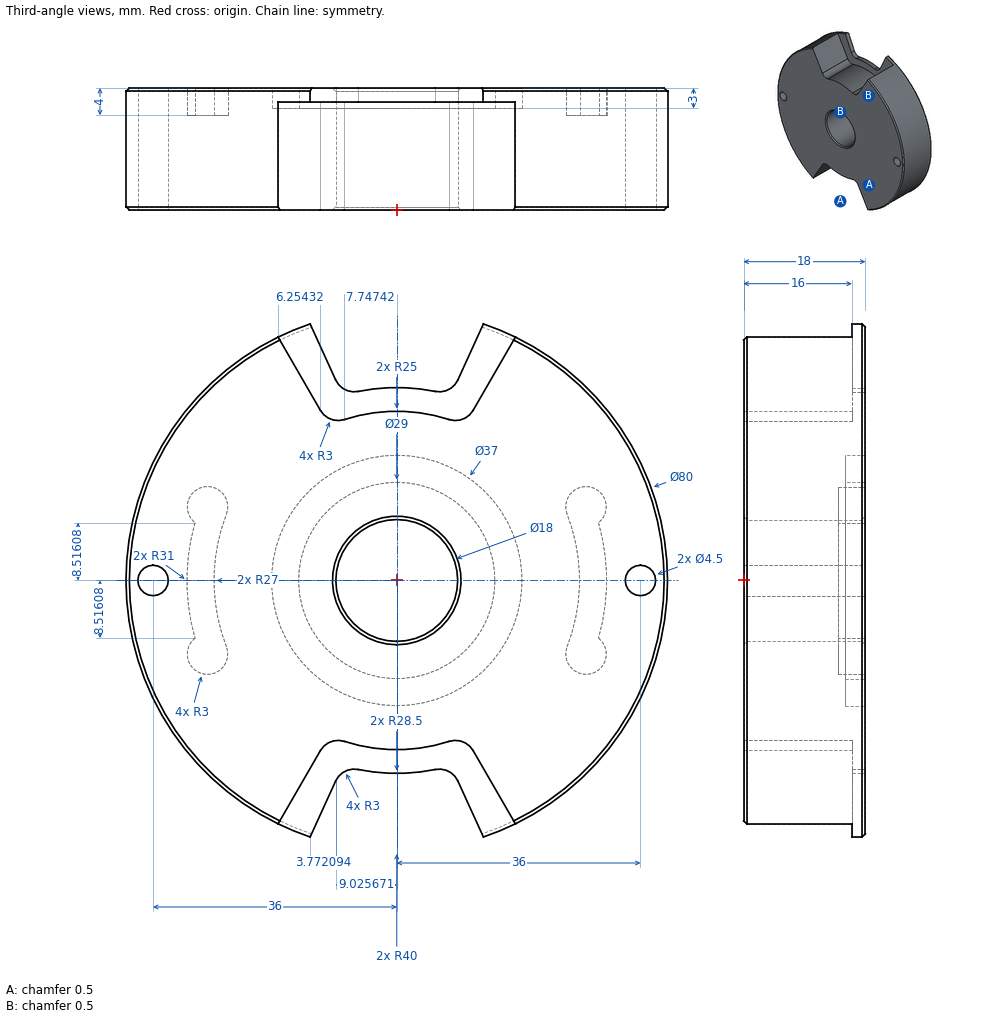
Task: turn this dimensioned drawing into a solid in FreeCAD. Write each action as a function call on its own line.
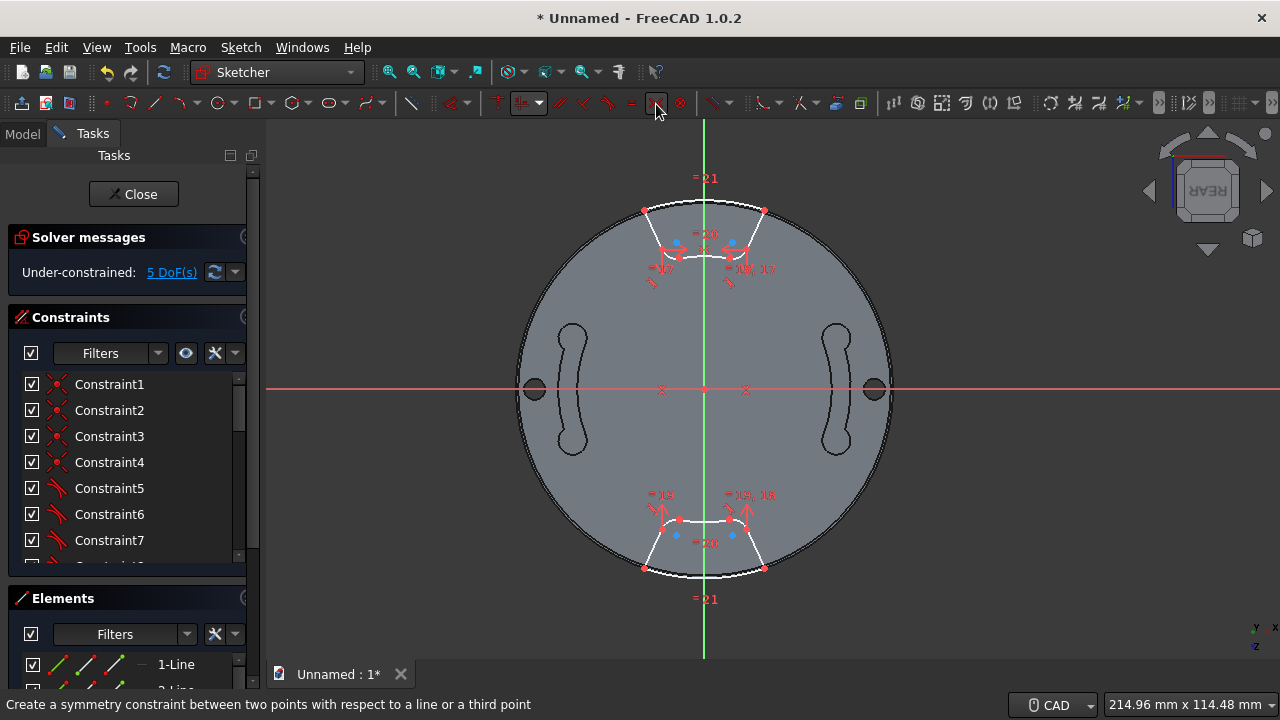
click(450, 104)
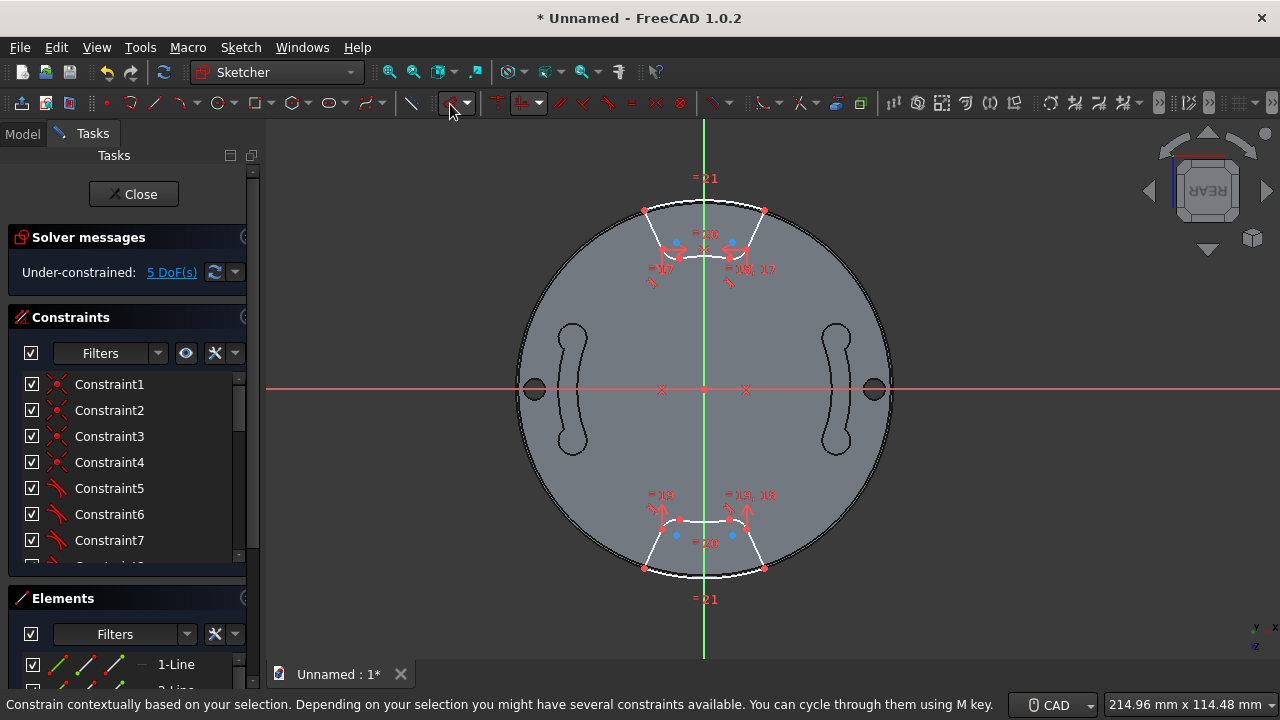
scroll(669, 257, up, 6)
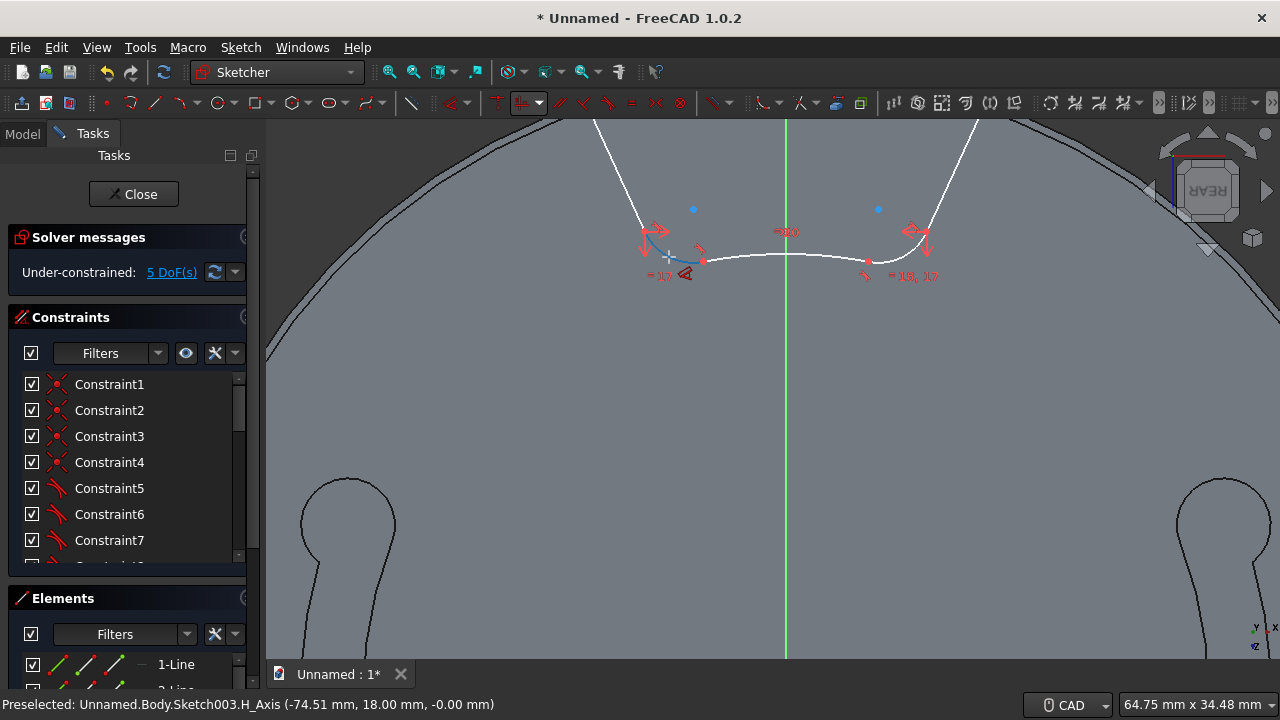
click(669, 257)
click(654, 285)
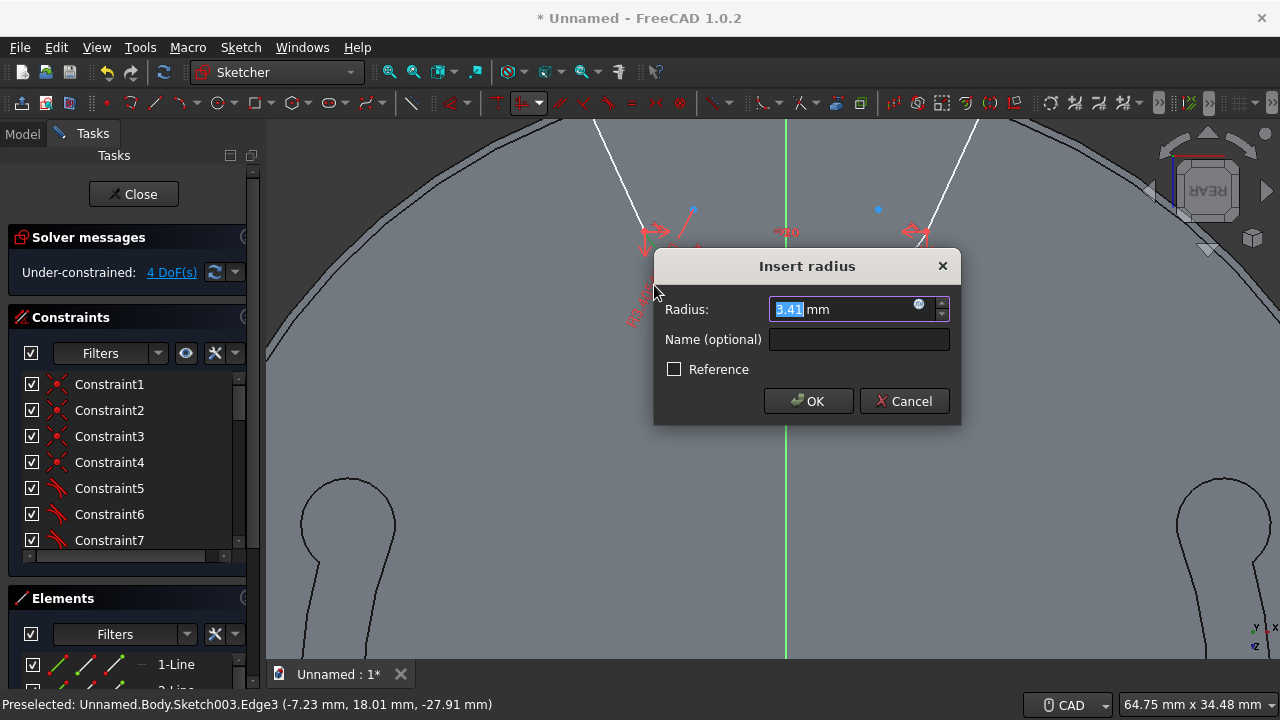
text(3)
key(Return)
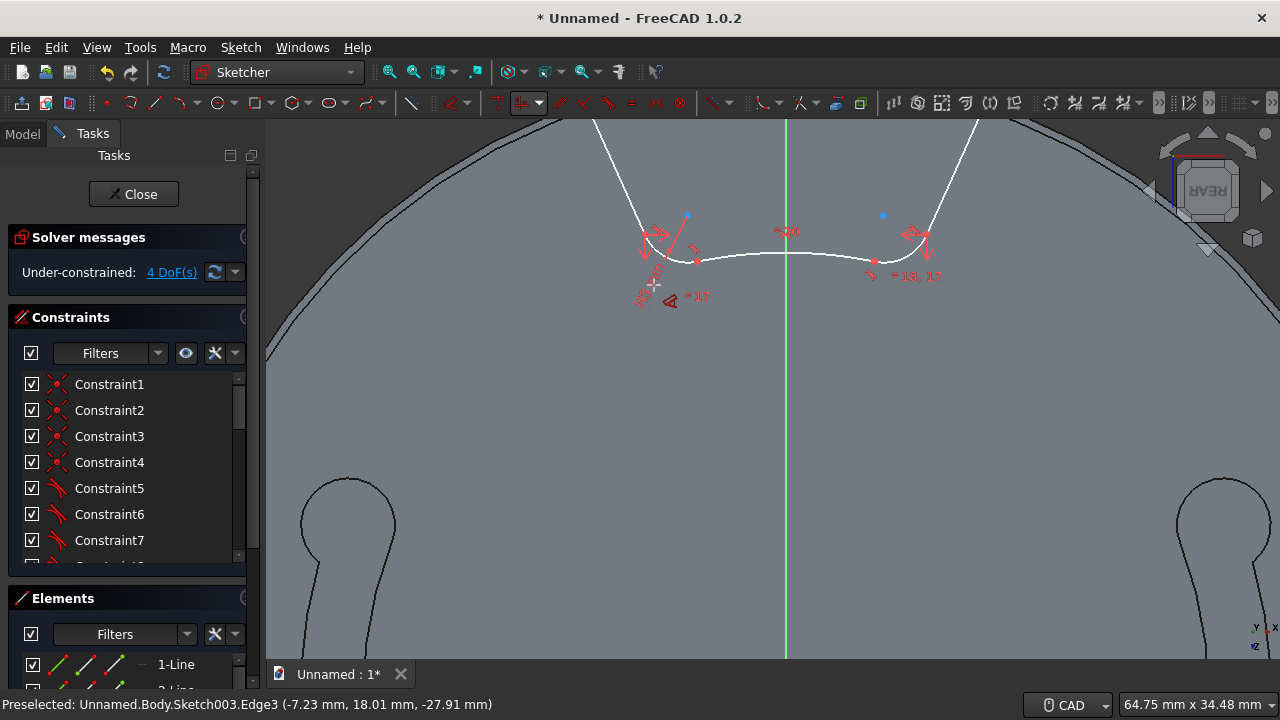
click(822, 254)
click(825, 222)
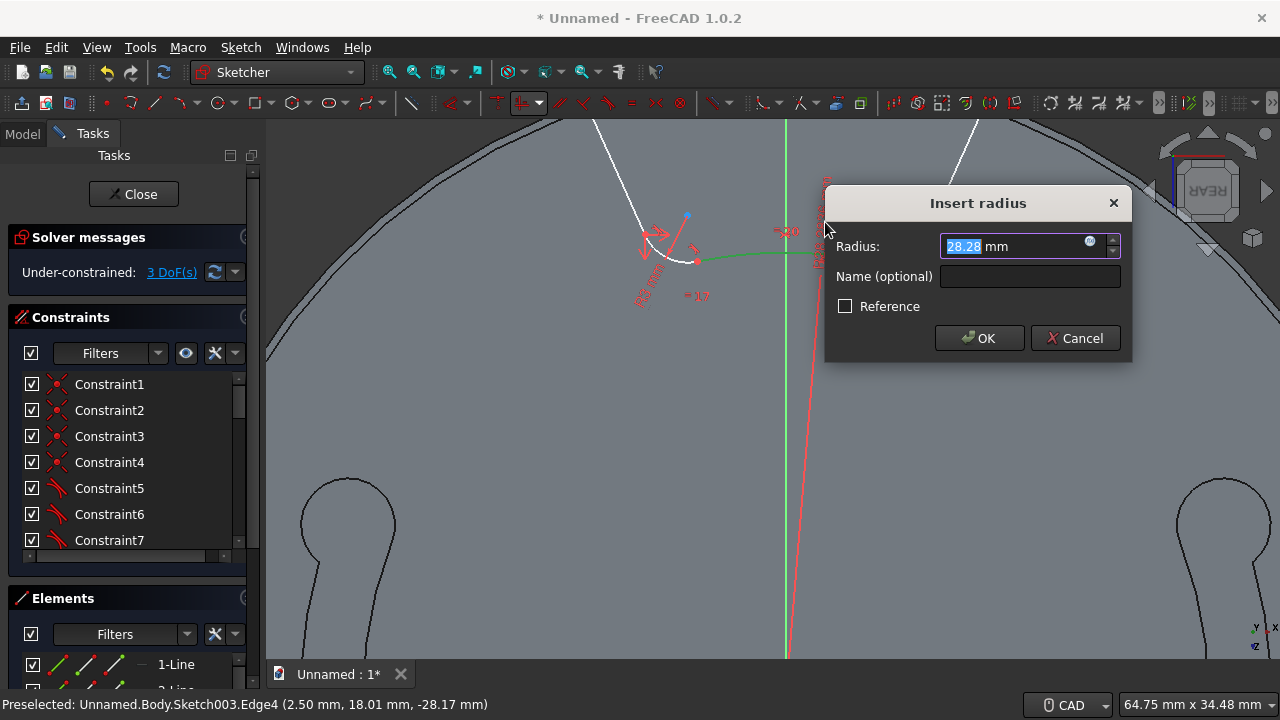
text(28.5)
key(Return)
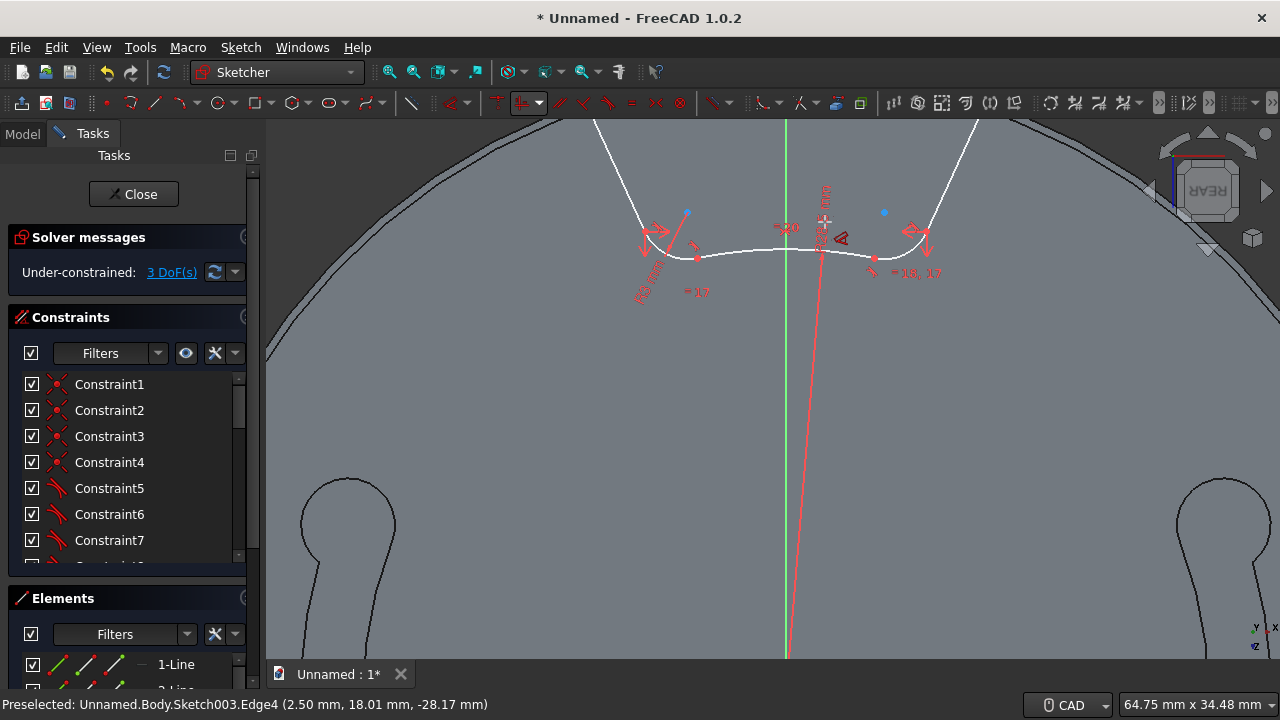
scroll(669, 257, down, 6)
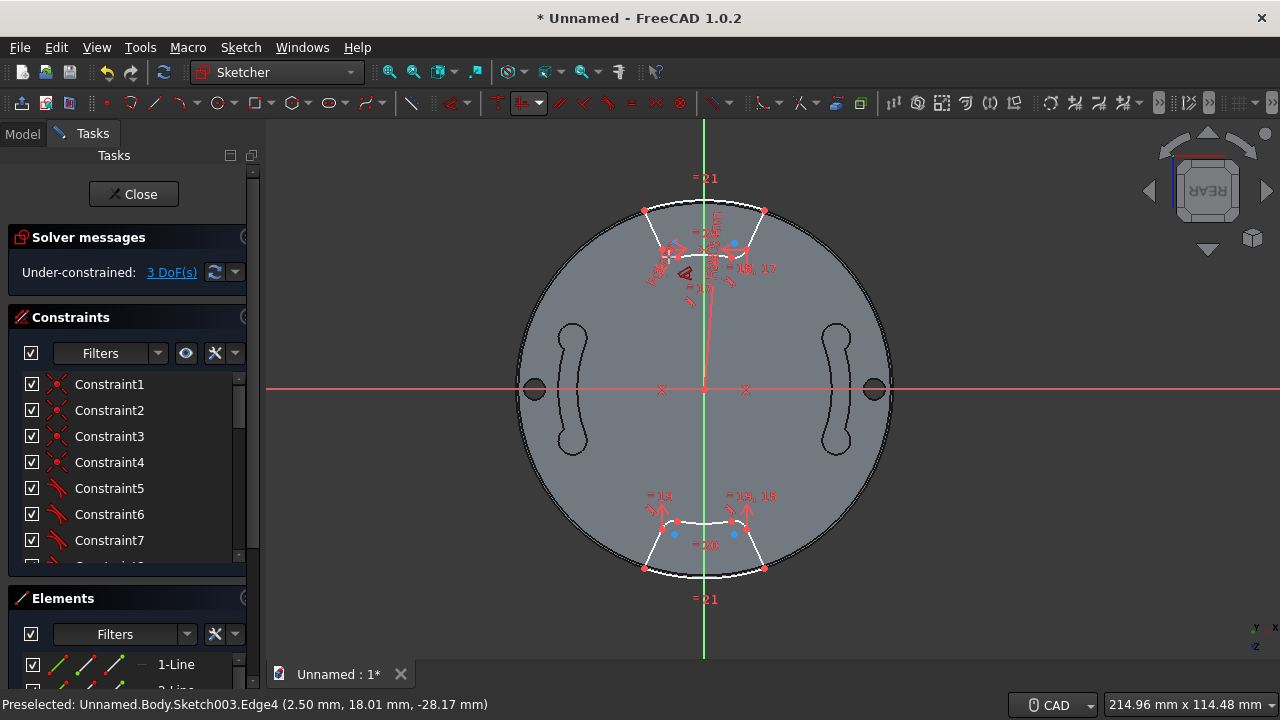
click(729, 202)
click(733, 170)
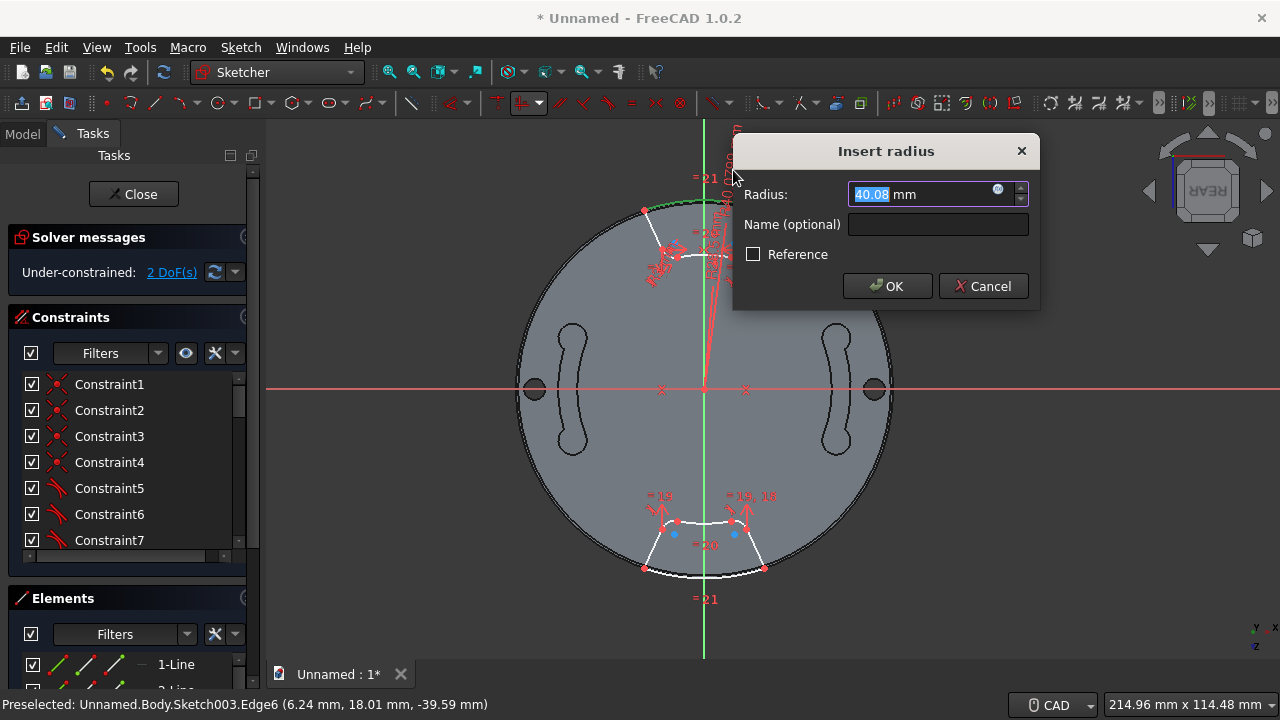
text(40)
key(Return)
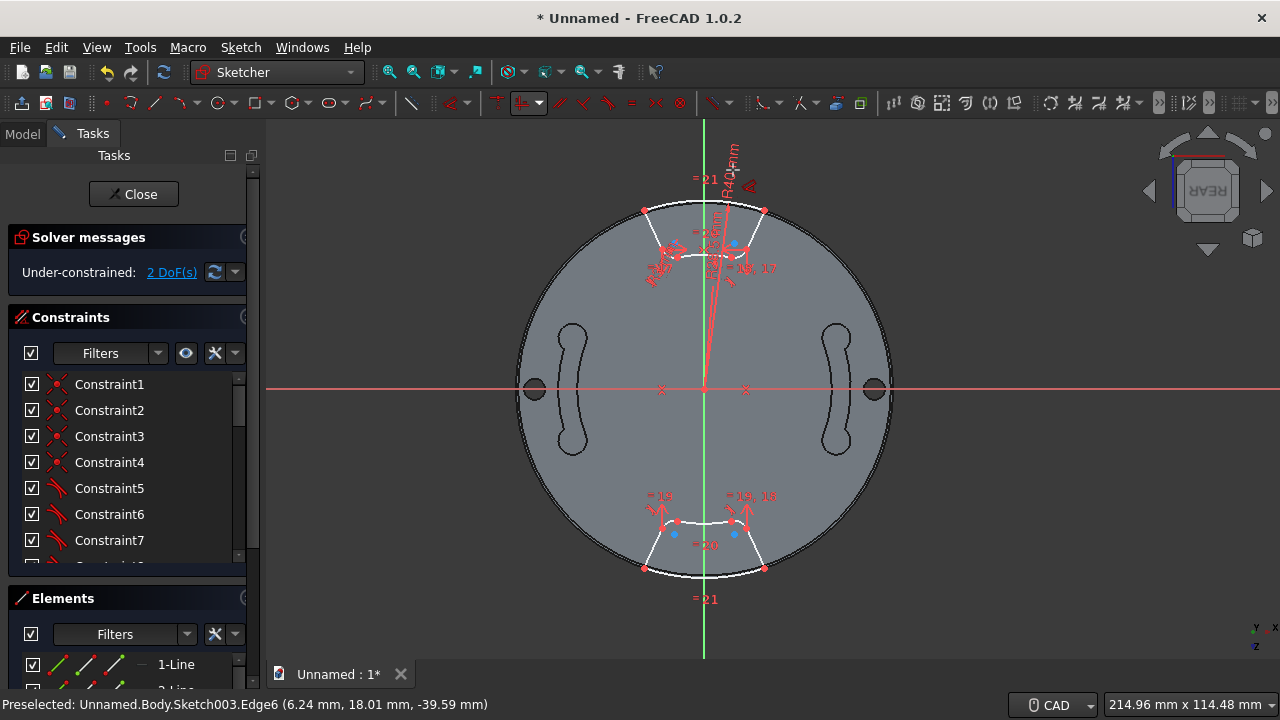
click(662, 250)
click(683, 216)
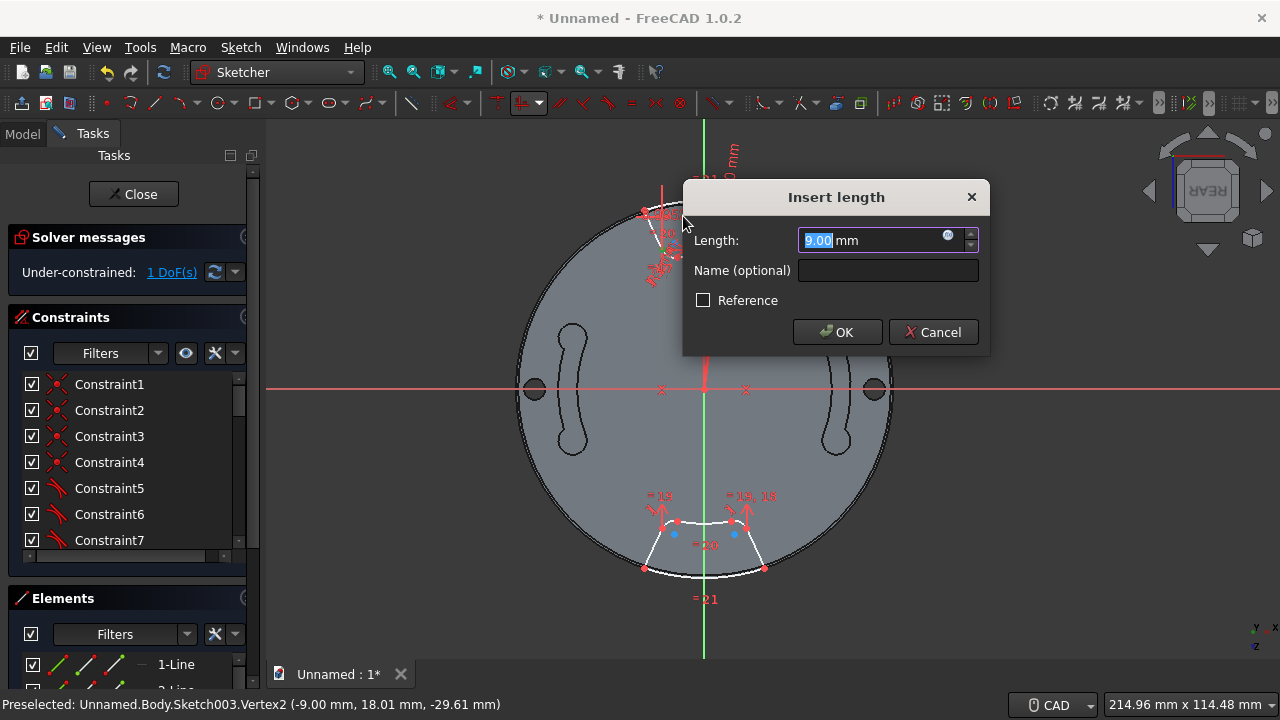
text(9.025671)
key(Return)